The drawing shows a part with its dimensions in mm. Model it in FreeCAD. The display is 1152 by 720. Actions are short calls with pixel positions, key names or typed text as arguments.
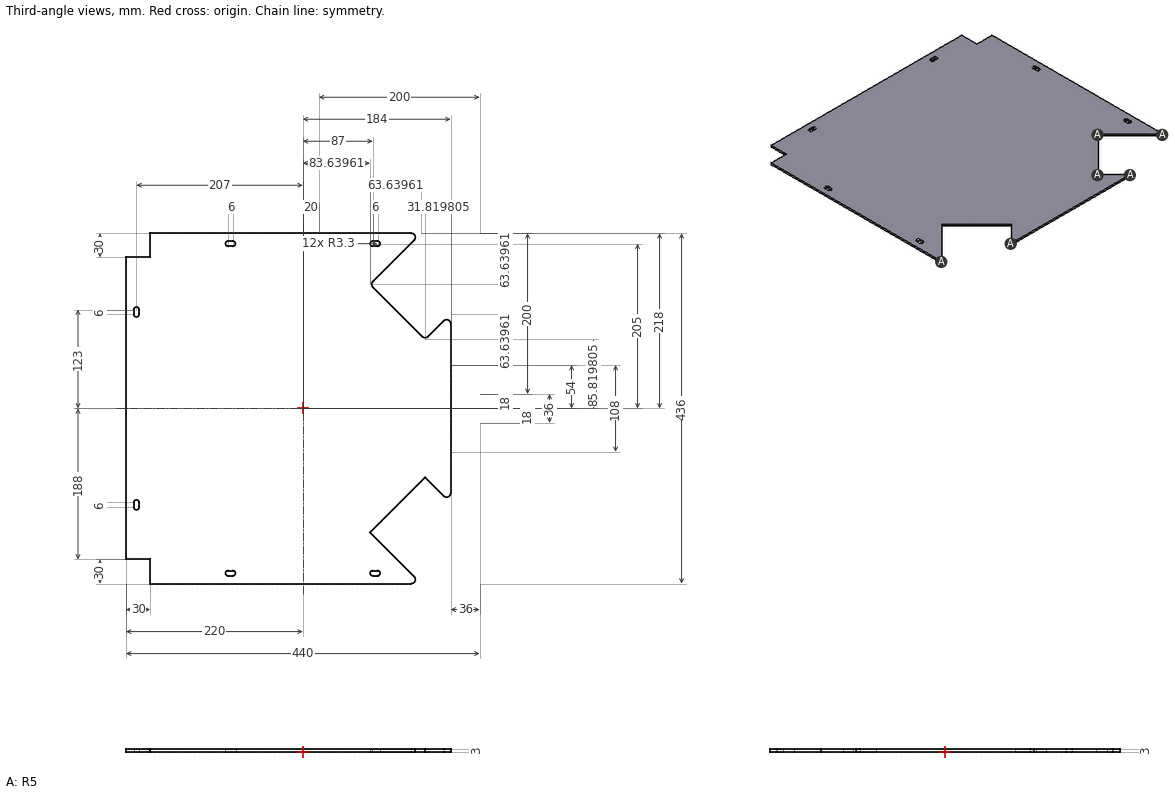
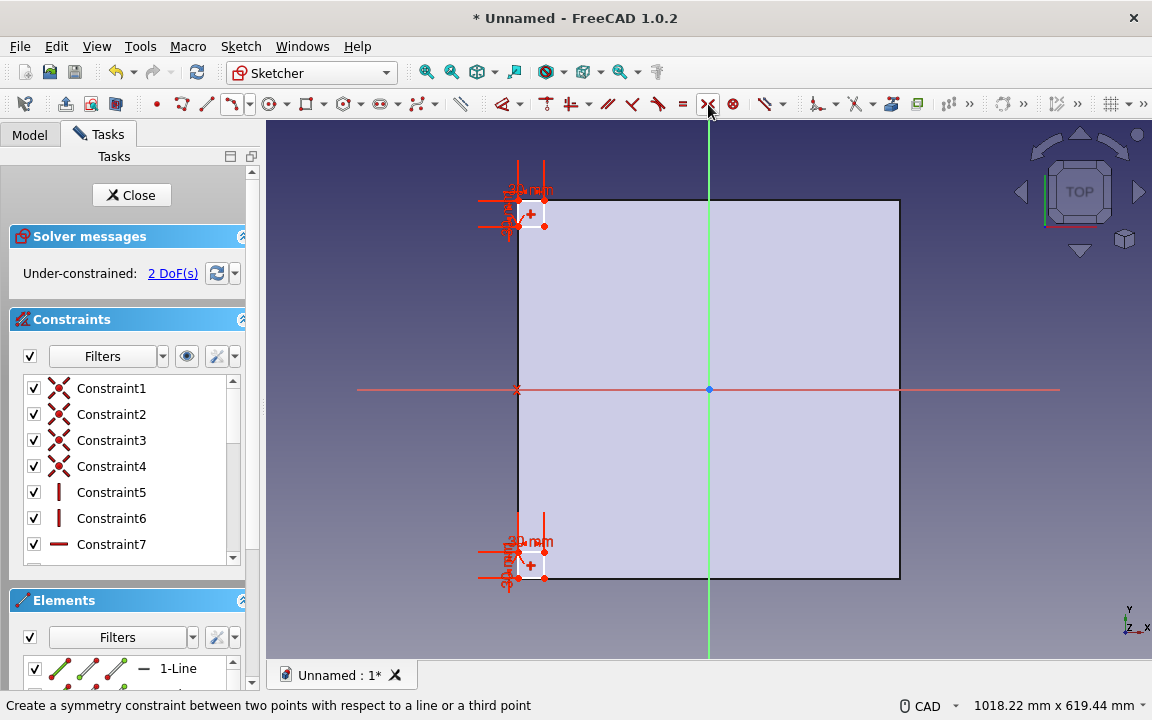
key(d)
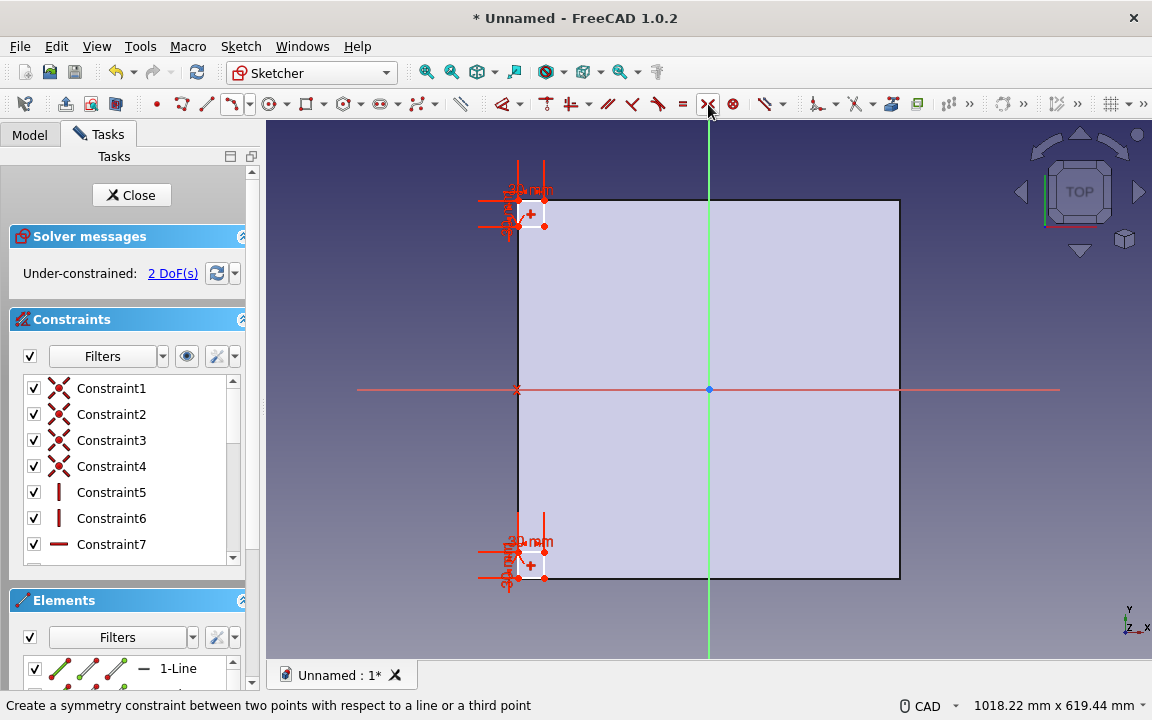
click(518, 552)
click(613, 586)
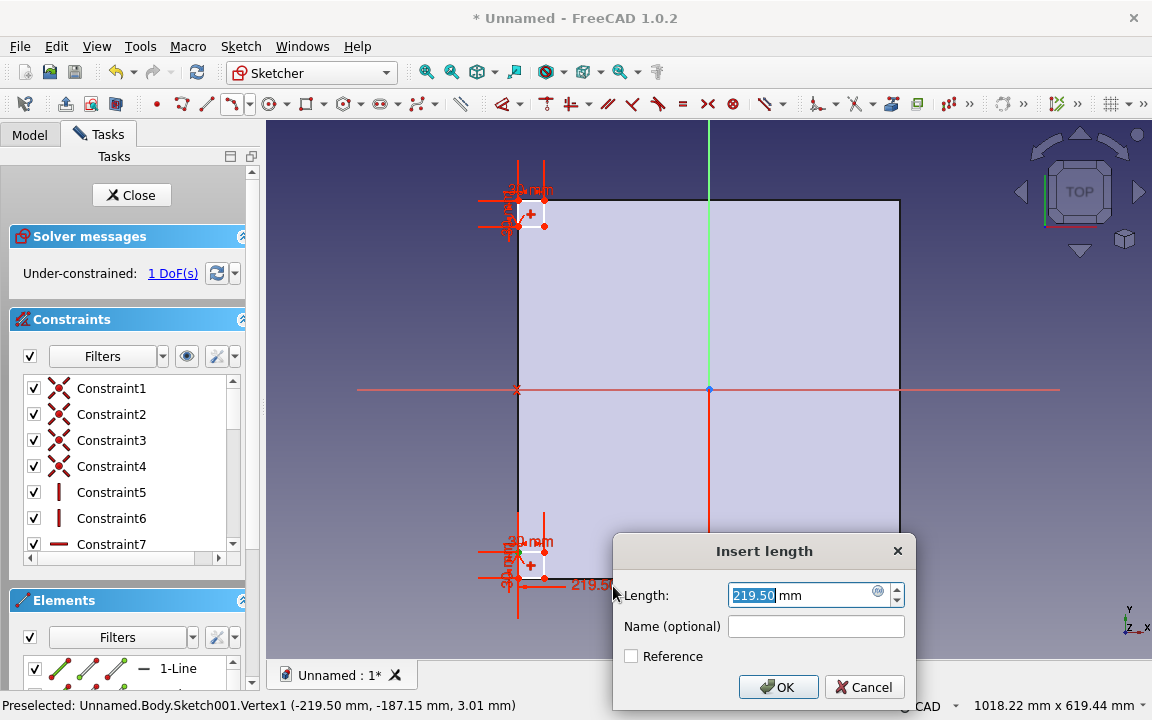
text(220)
key(Return)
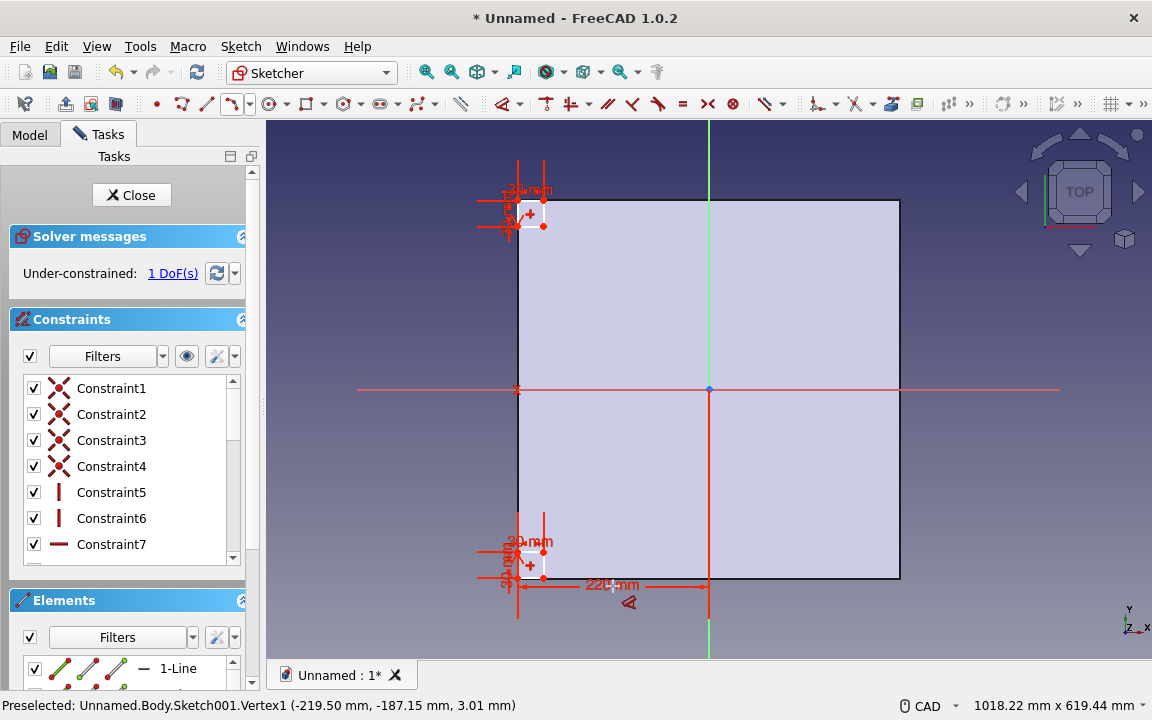
click(518, 552)
click(743, 471)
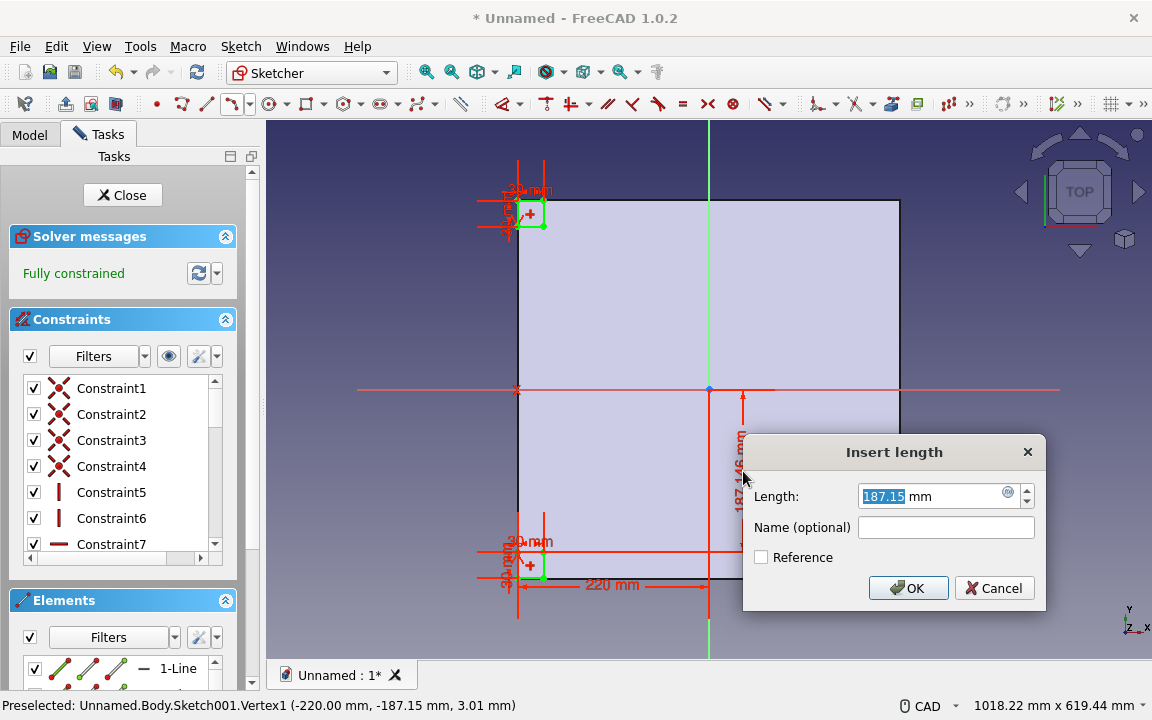
text(188)
key(Return)
key(Escape)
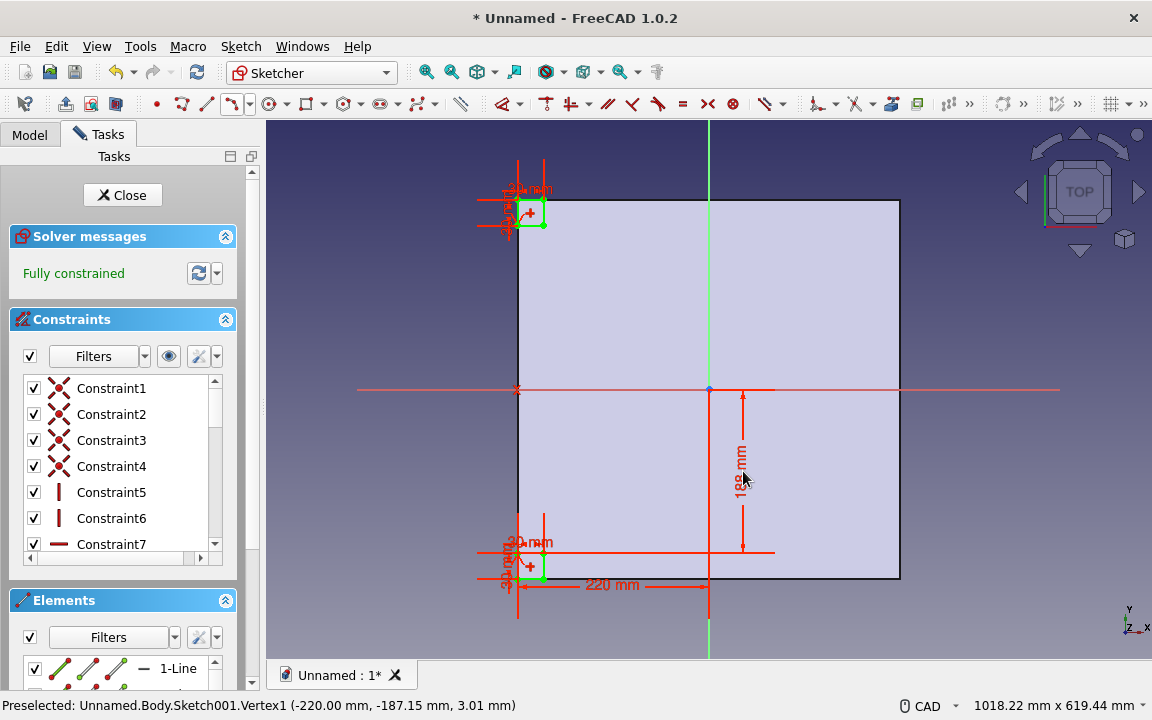
click(123, 195)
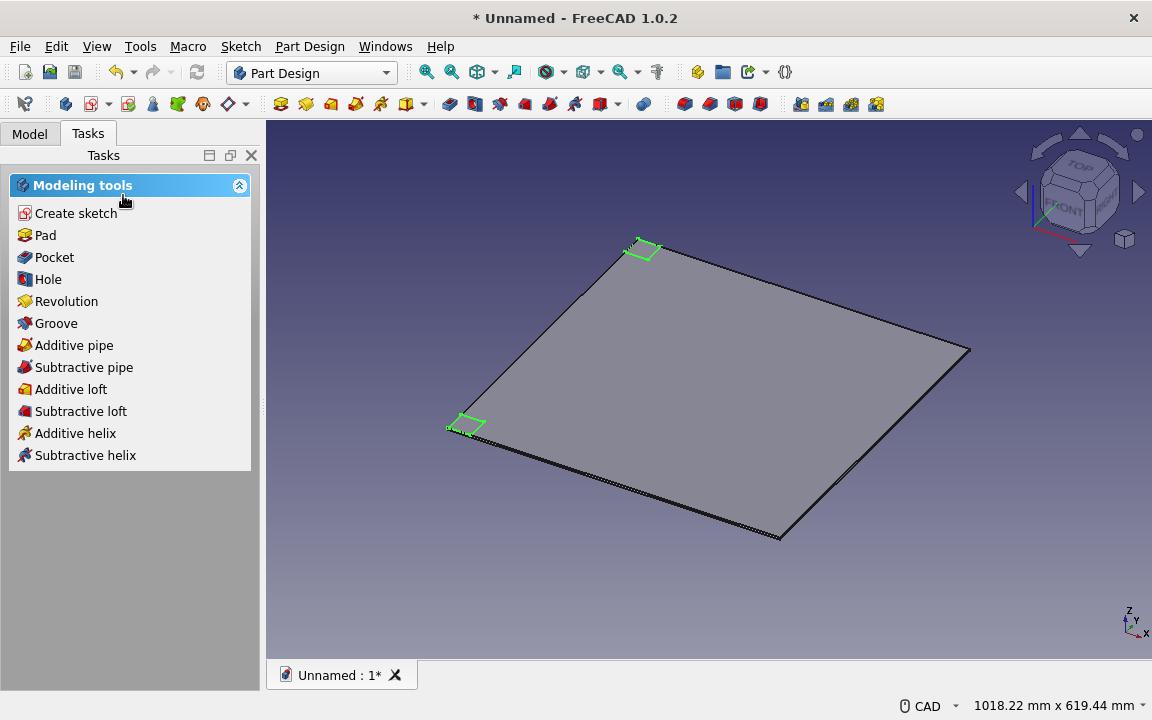
click(450, 104)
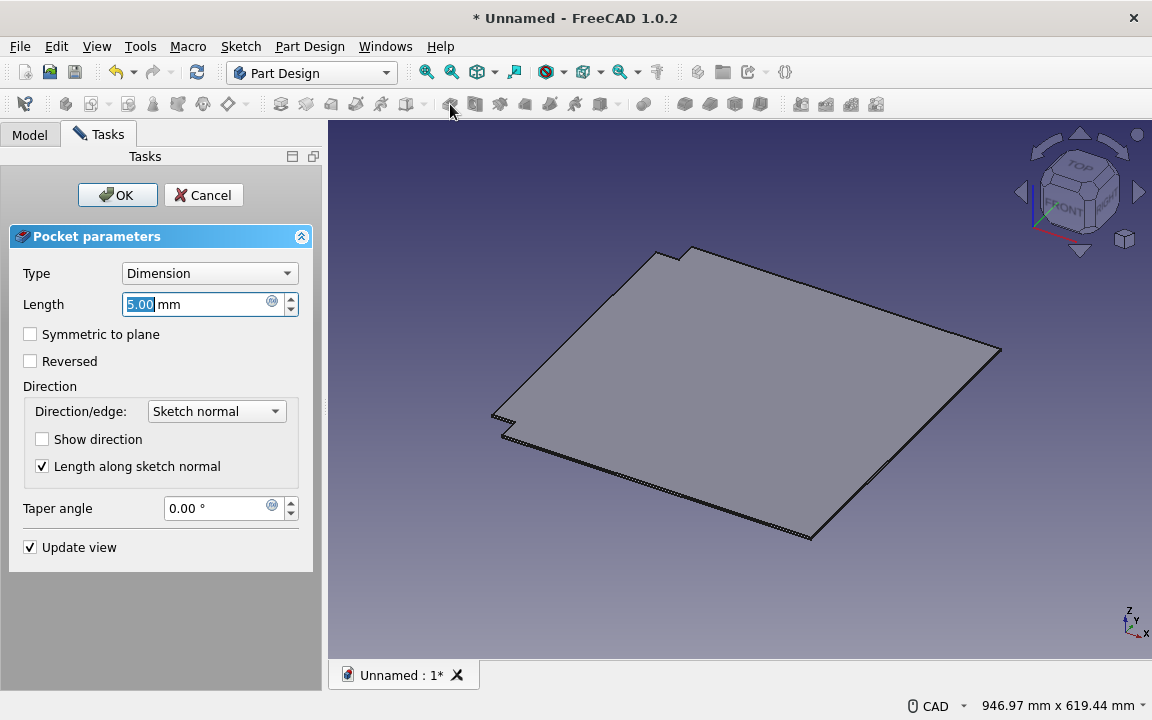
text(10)
key(Tab)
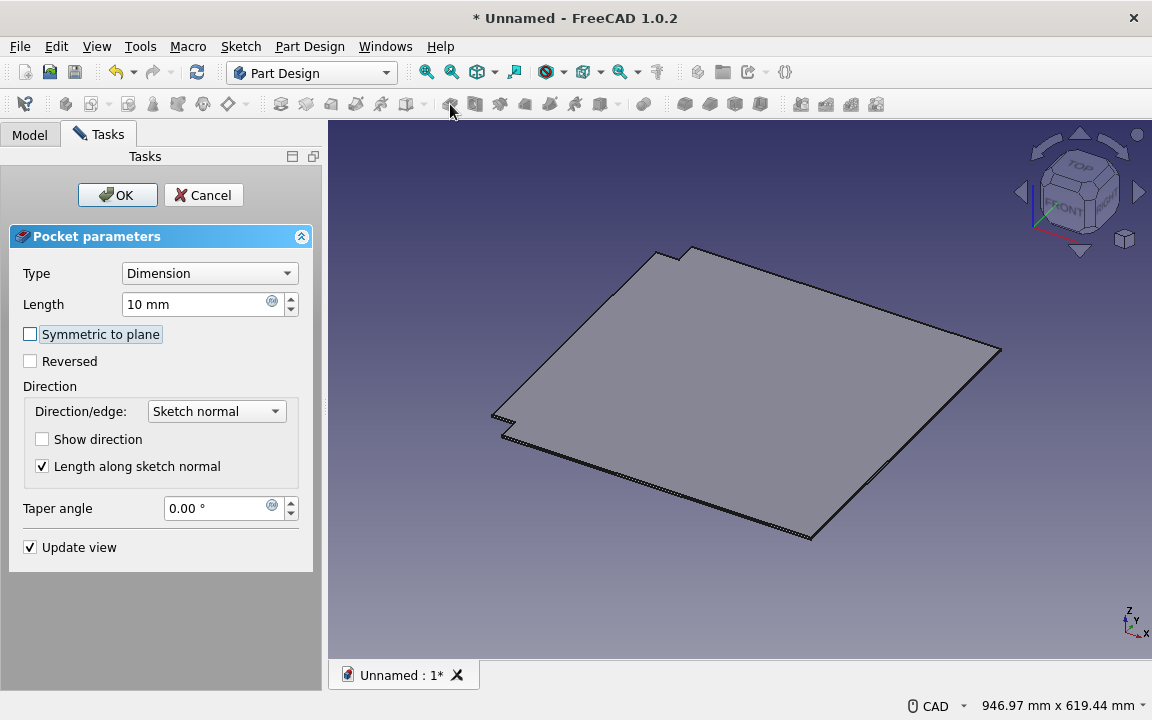
click(118, 195)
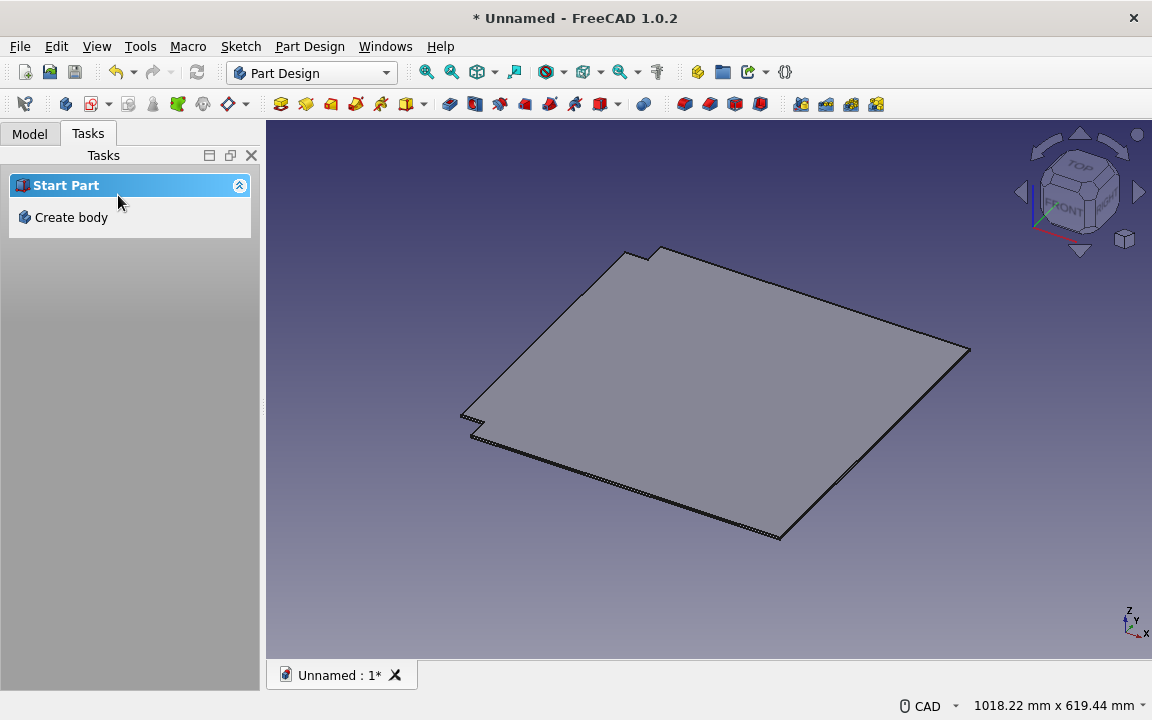
click(709, 387)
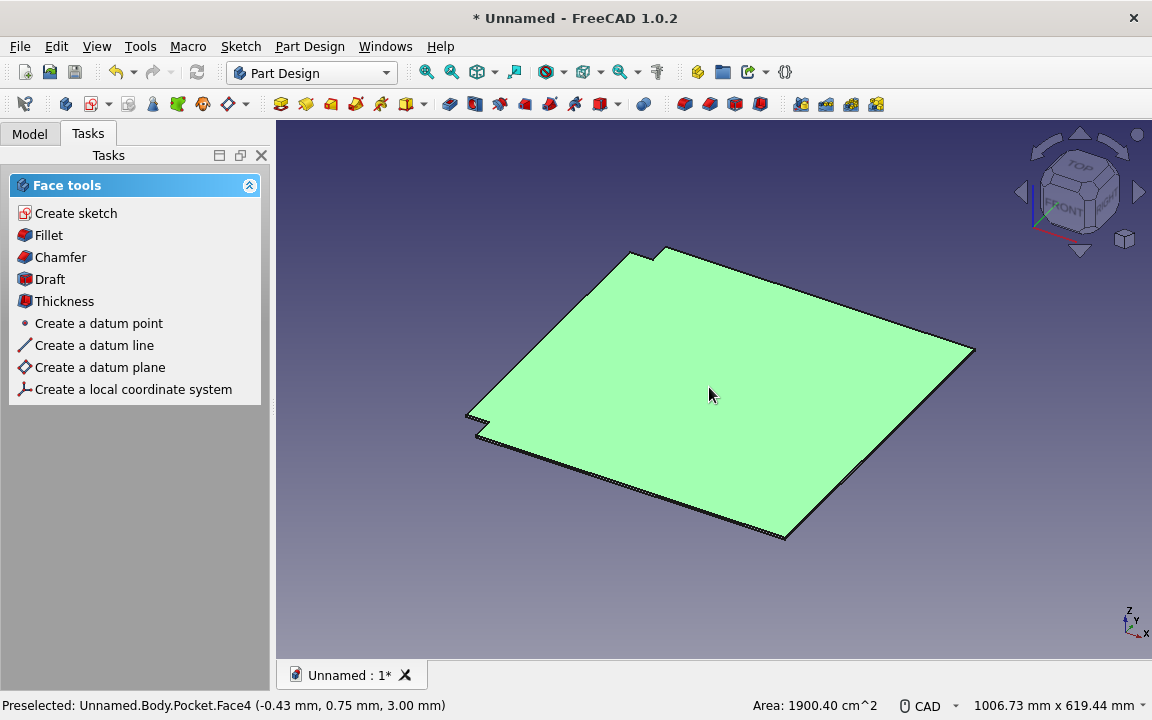
click(90, 104)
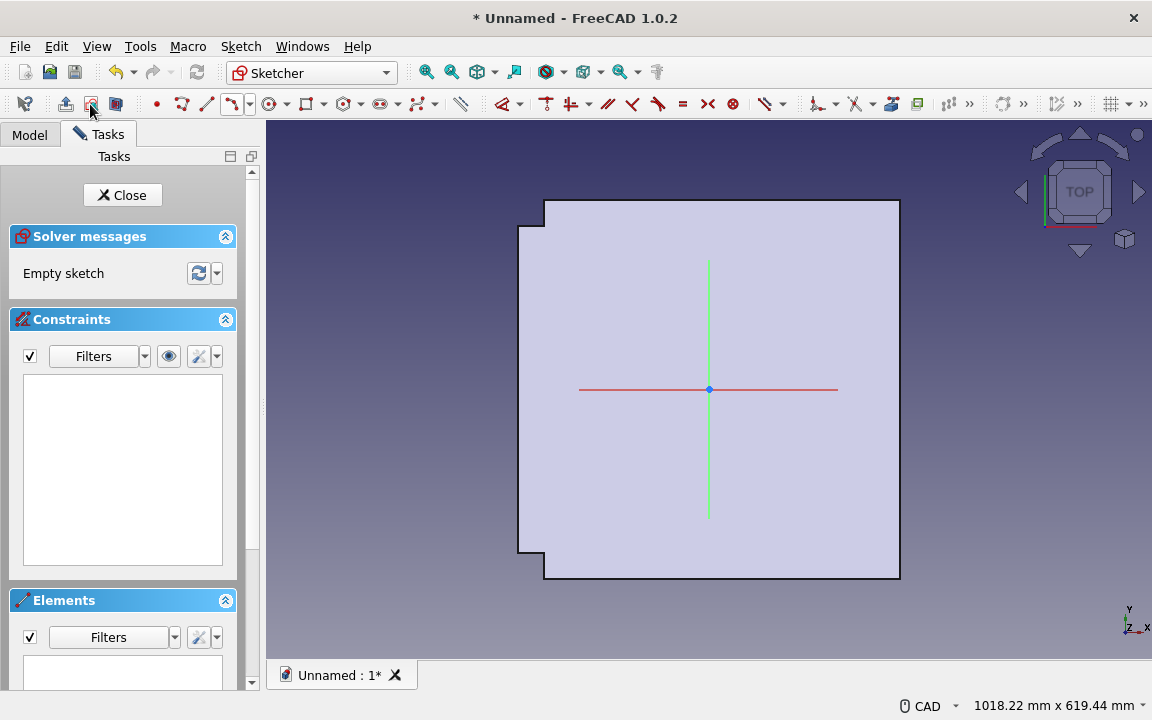
click(182, 104)